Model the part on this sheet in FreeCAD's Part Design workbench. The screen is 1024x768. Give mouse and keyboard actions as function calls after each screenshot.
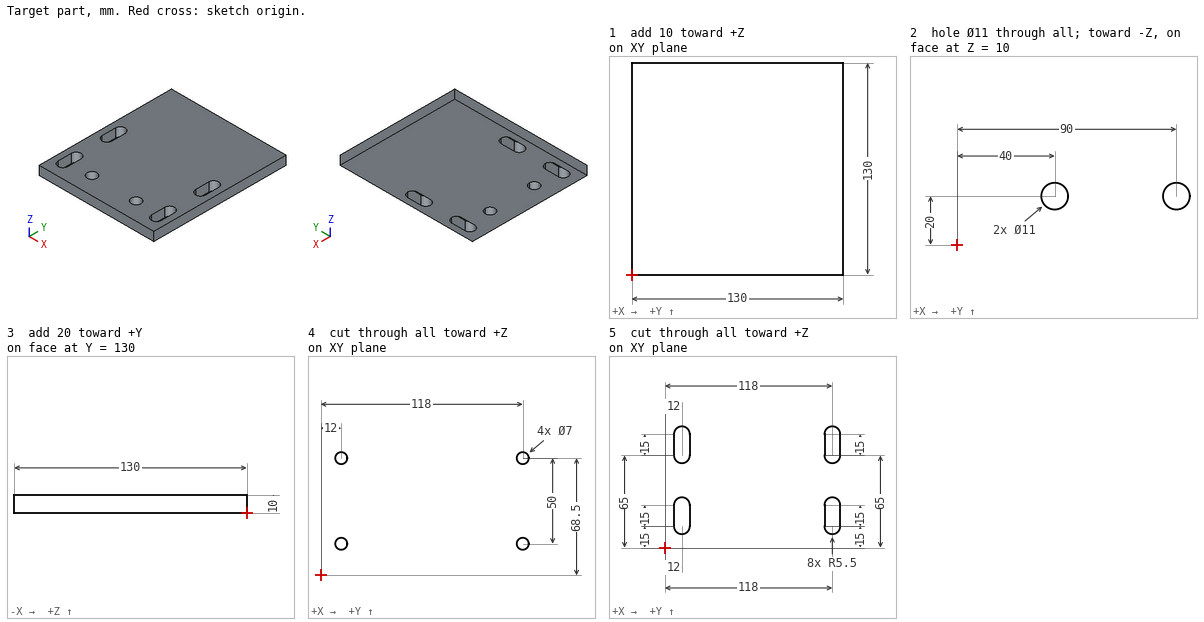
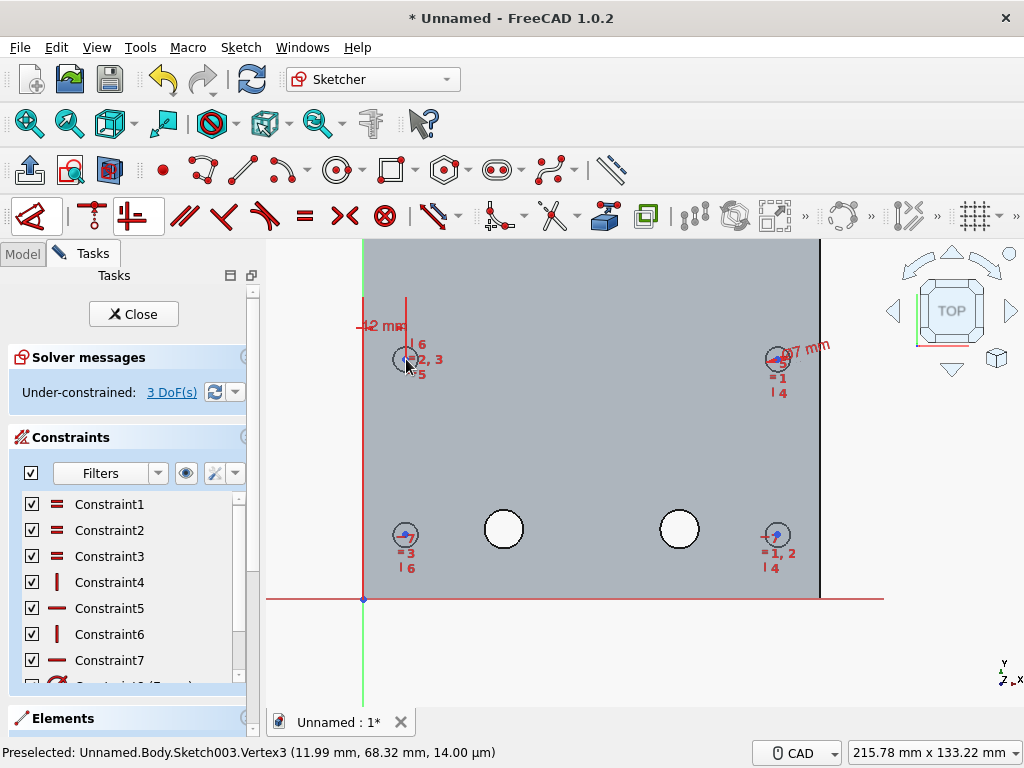
click(778, 359)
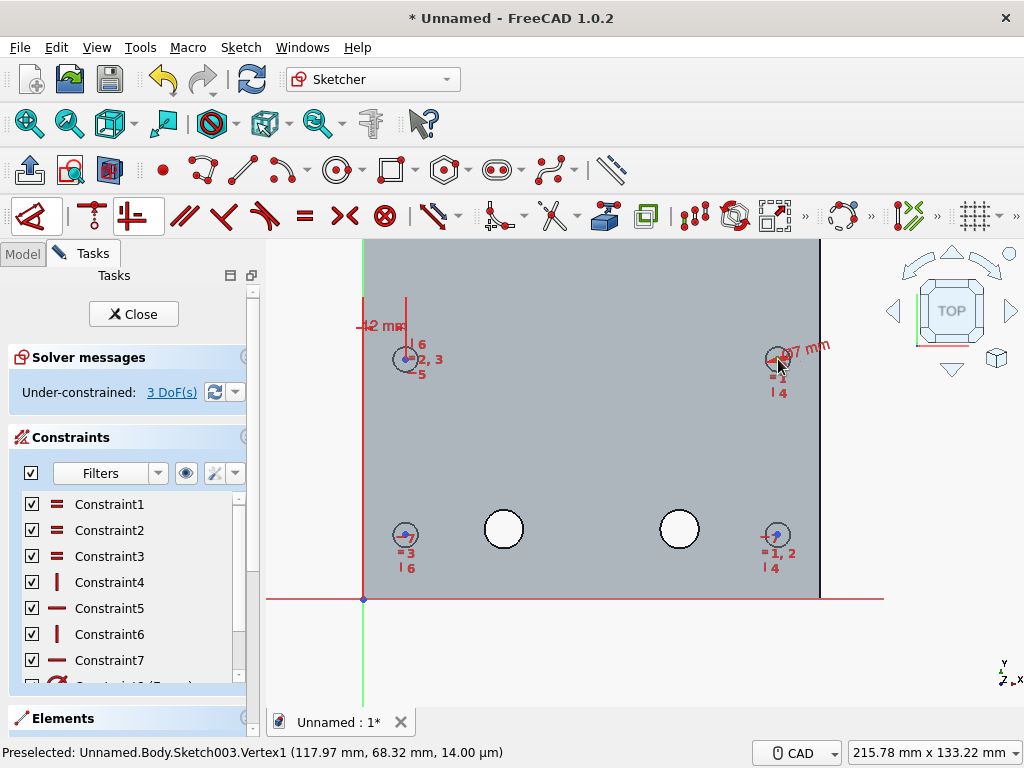
click(56, 216)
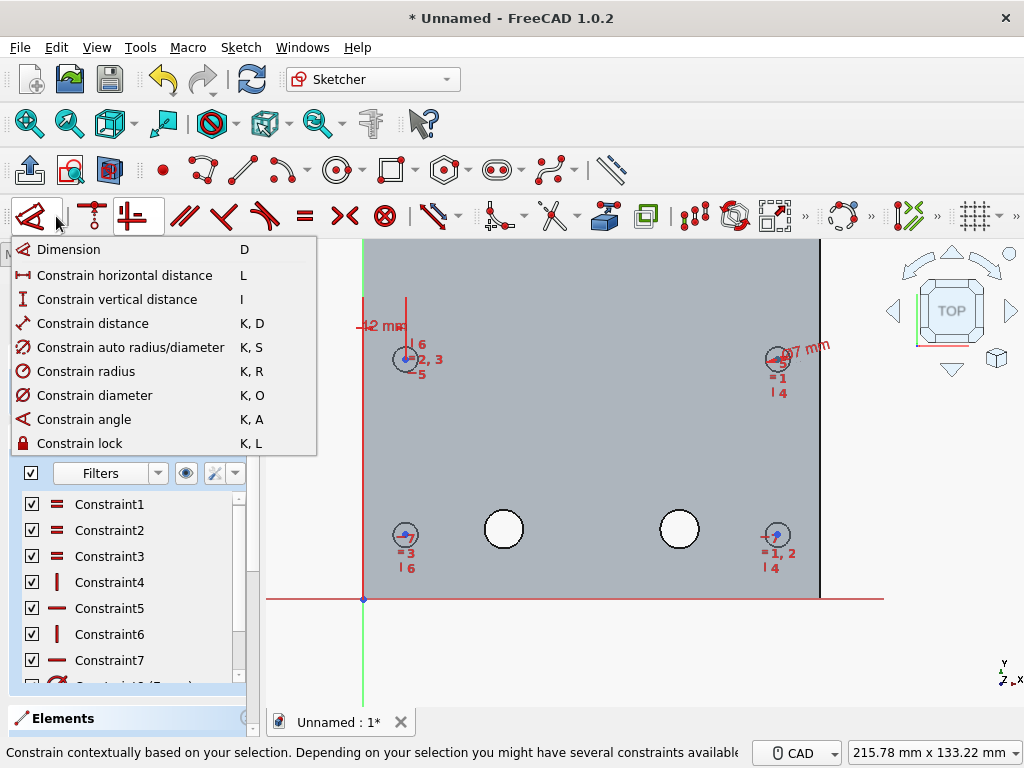
click(164, 275)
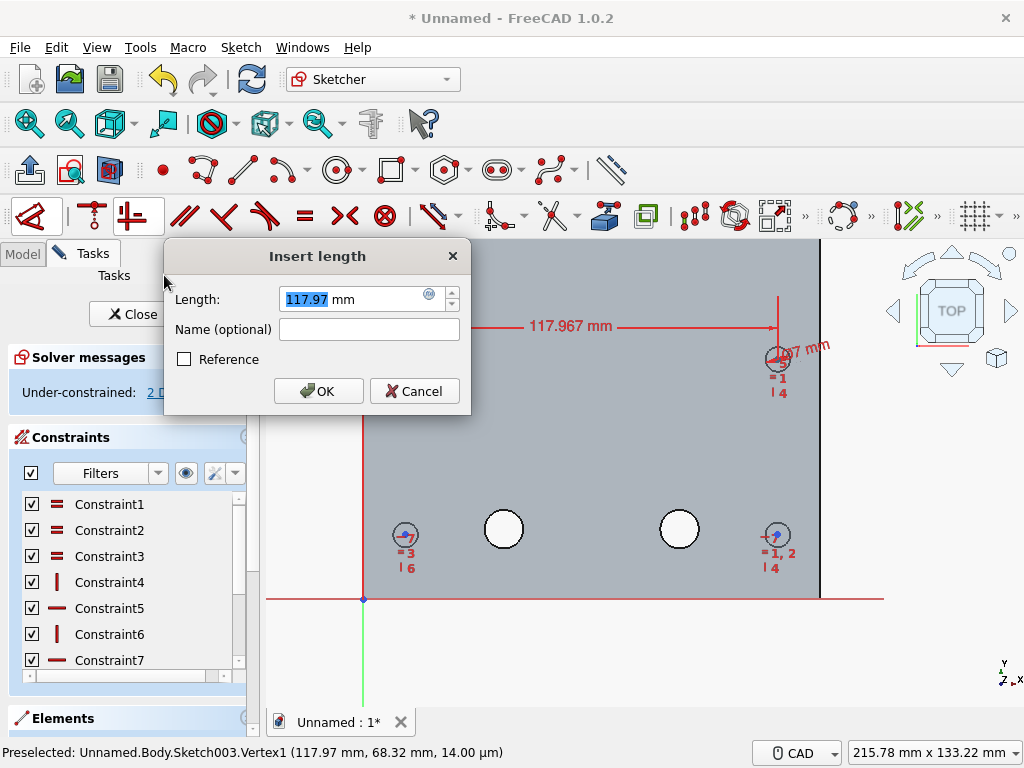
text(118)
key(Return)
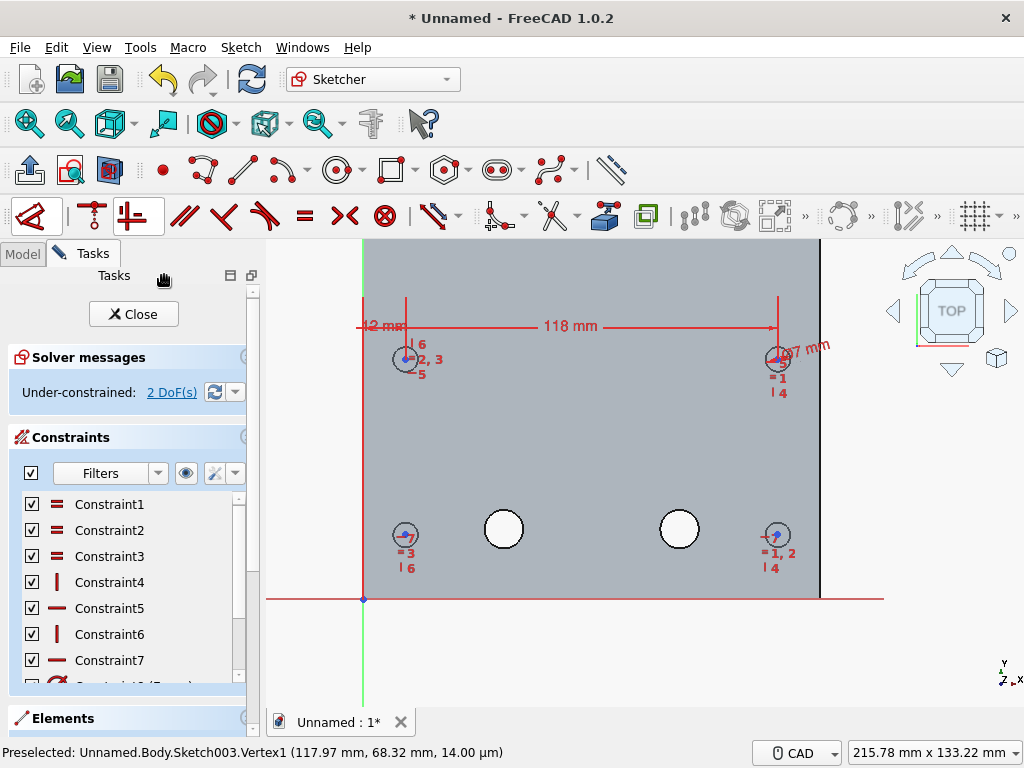
click(778, 359)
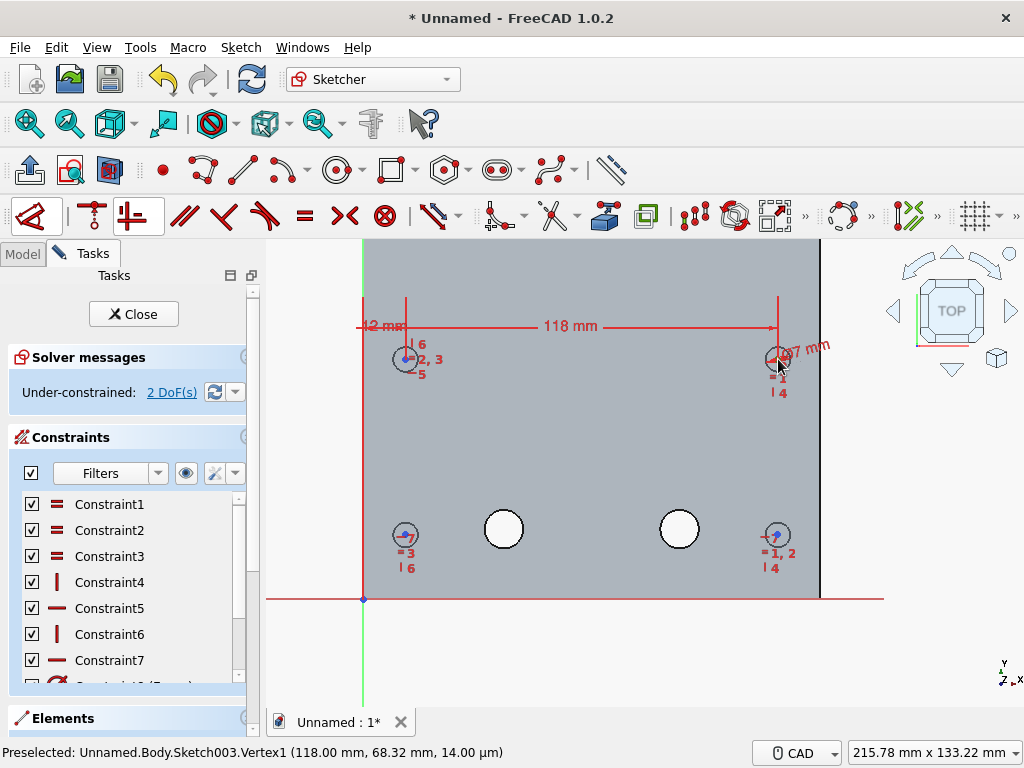
click(778, 535)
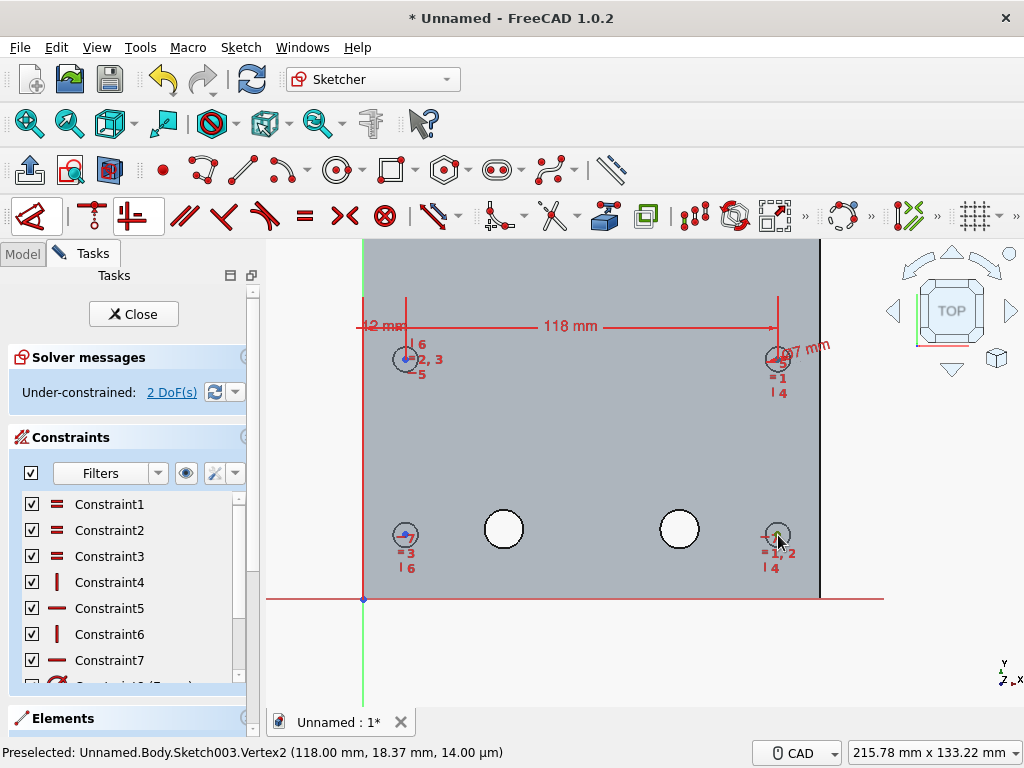
click(56, 216)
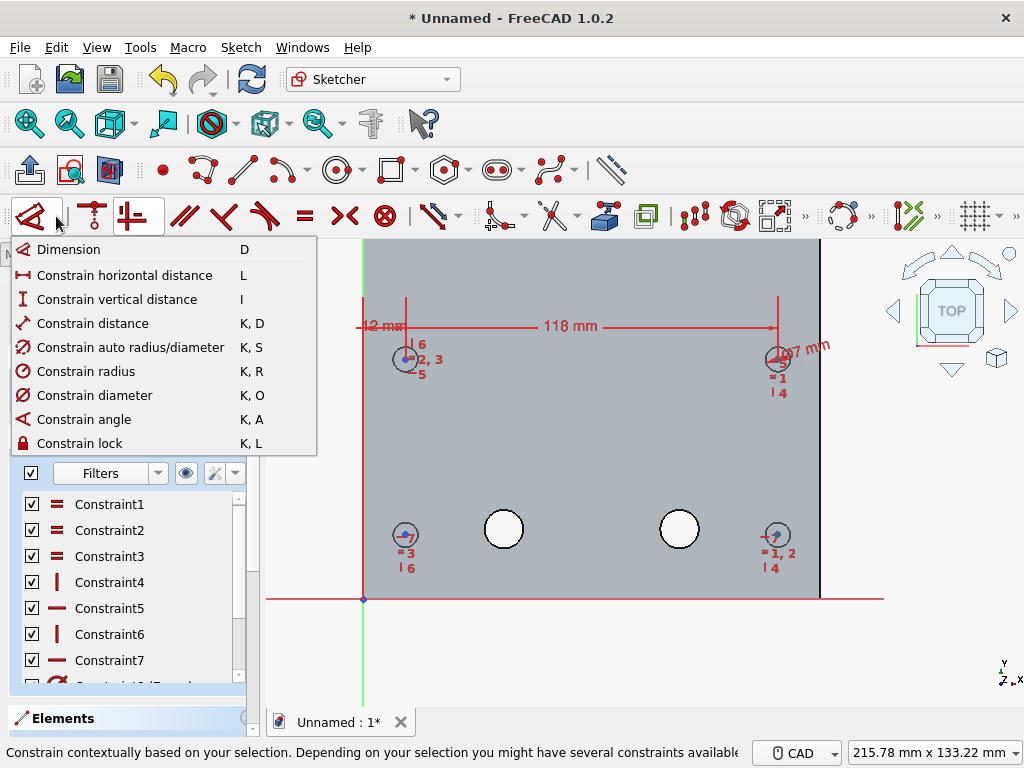
click(164, 299)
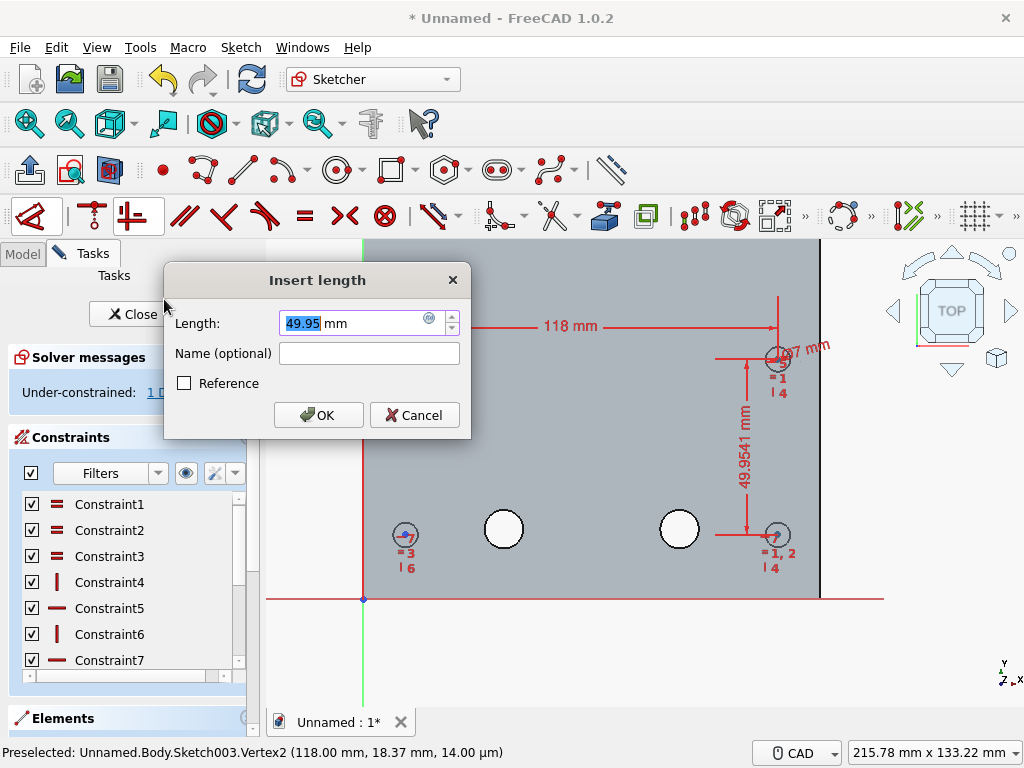
text(50)
key(Return)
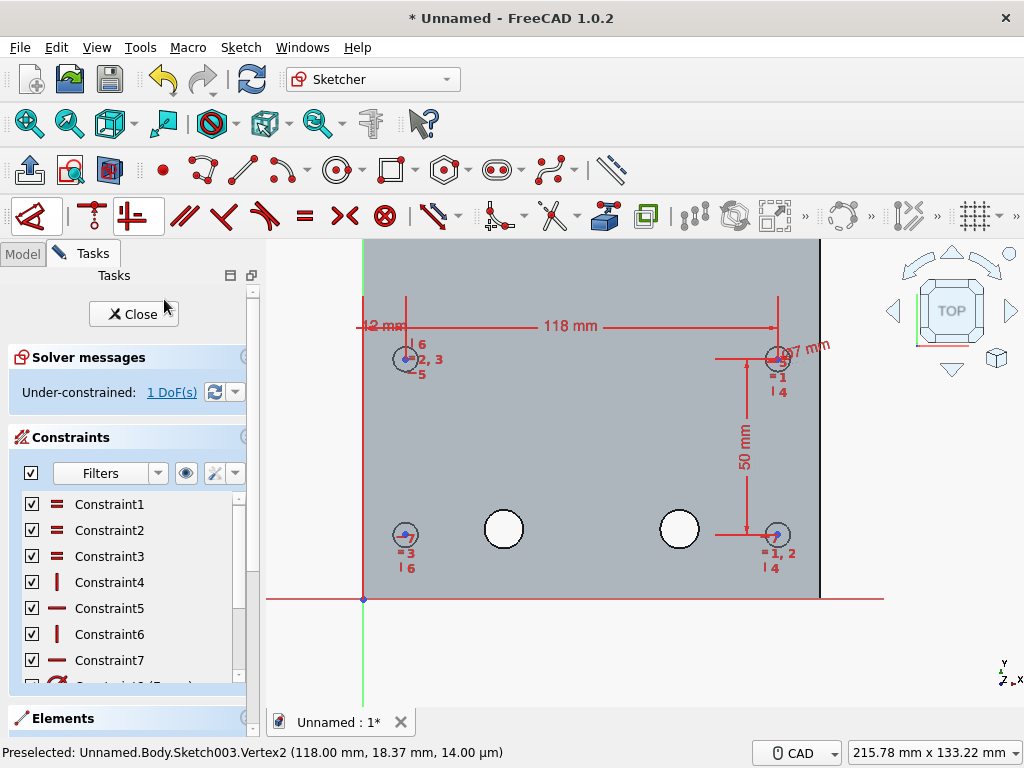
click(778, 359)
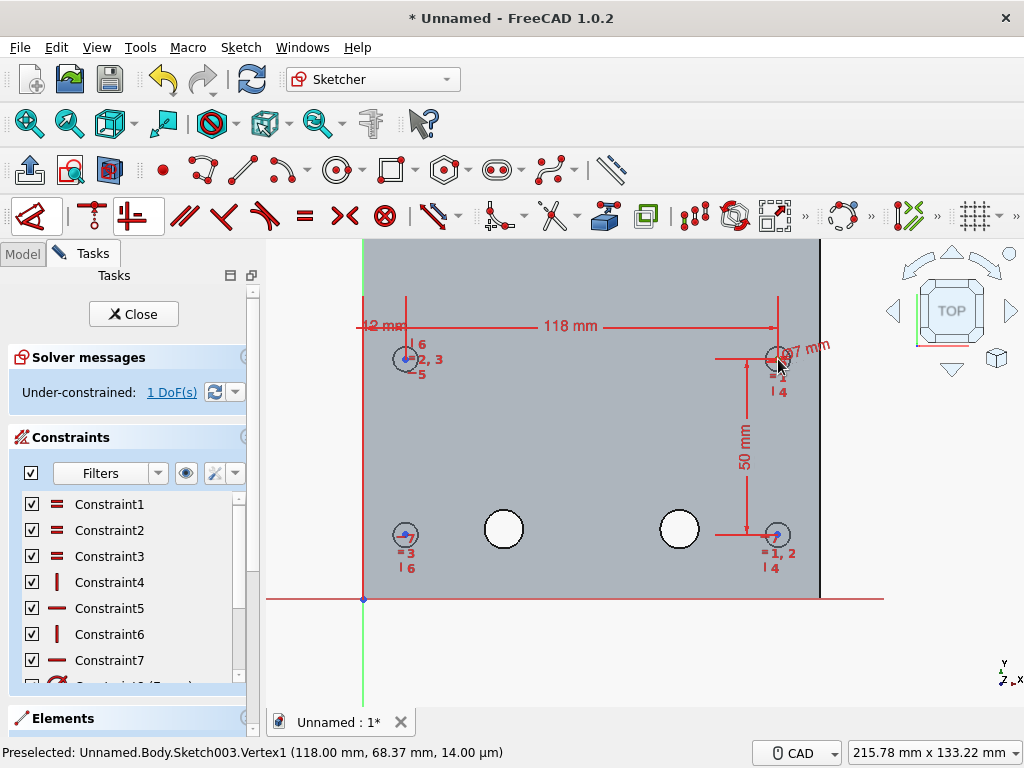
click(56, 216)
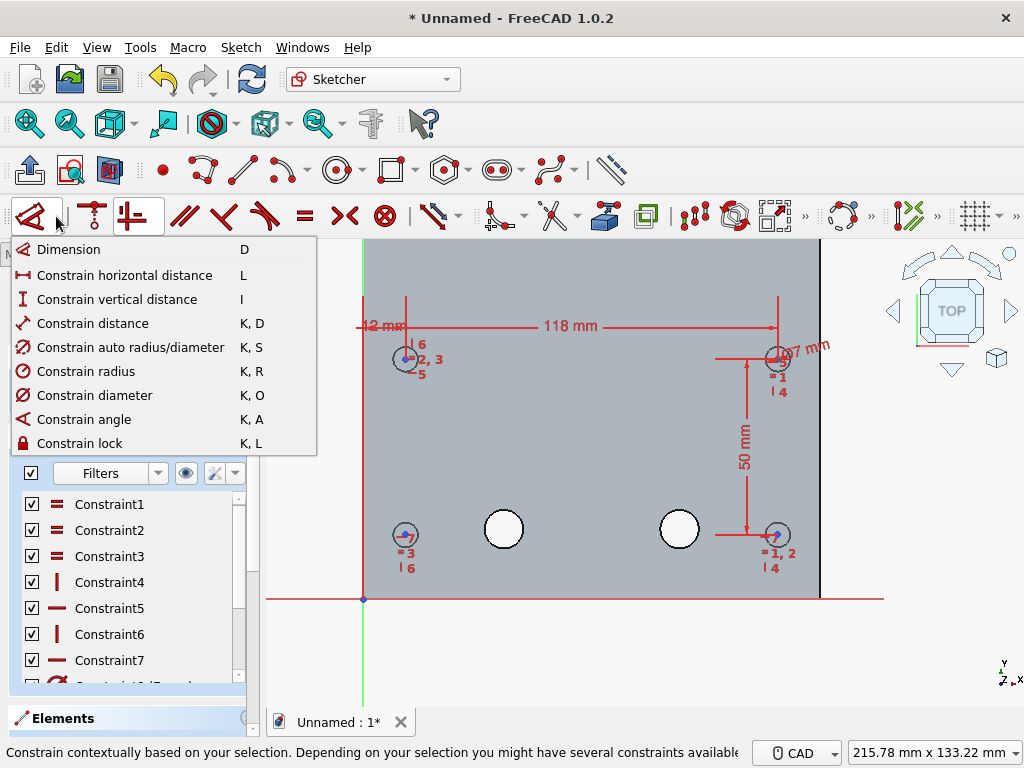
click(164, 299)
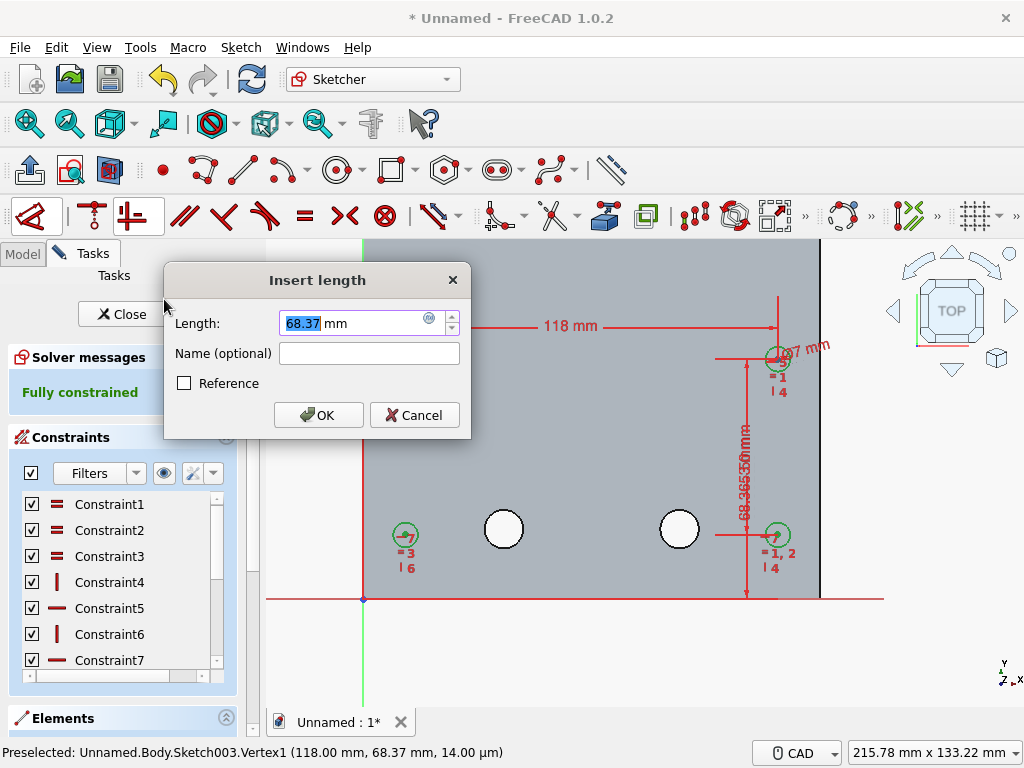
text(68.5)
key(Return)